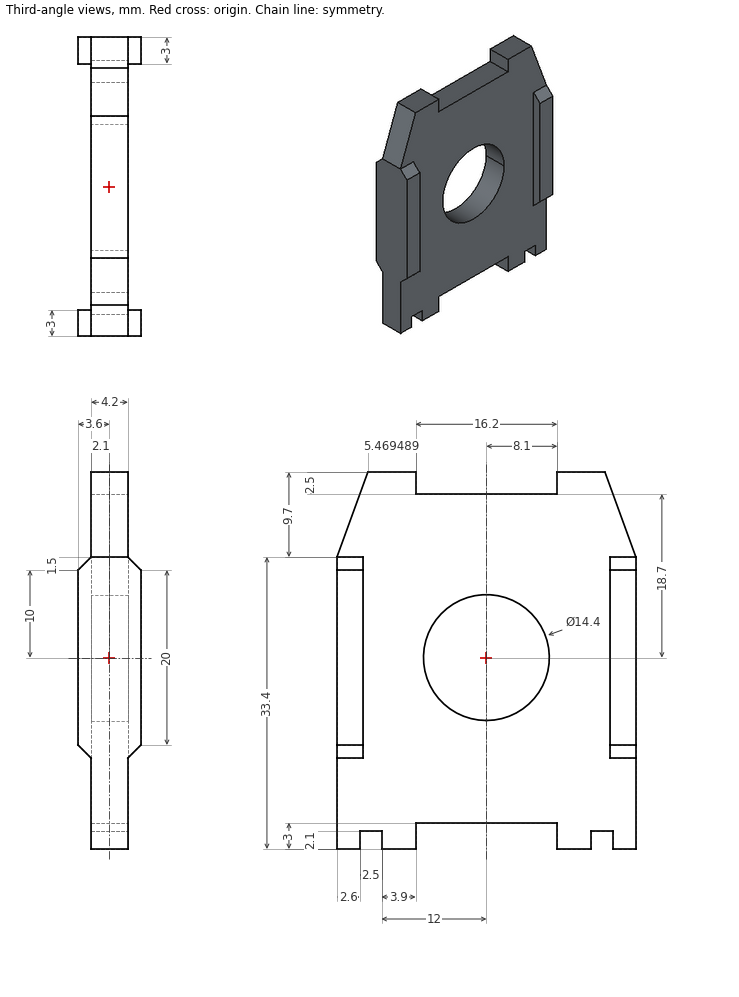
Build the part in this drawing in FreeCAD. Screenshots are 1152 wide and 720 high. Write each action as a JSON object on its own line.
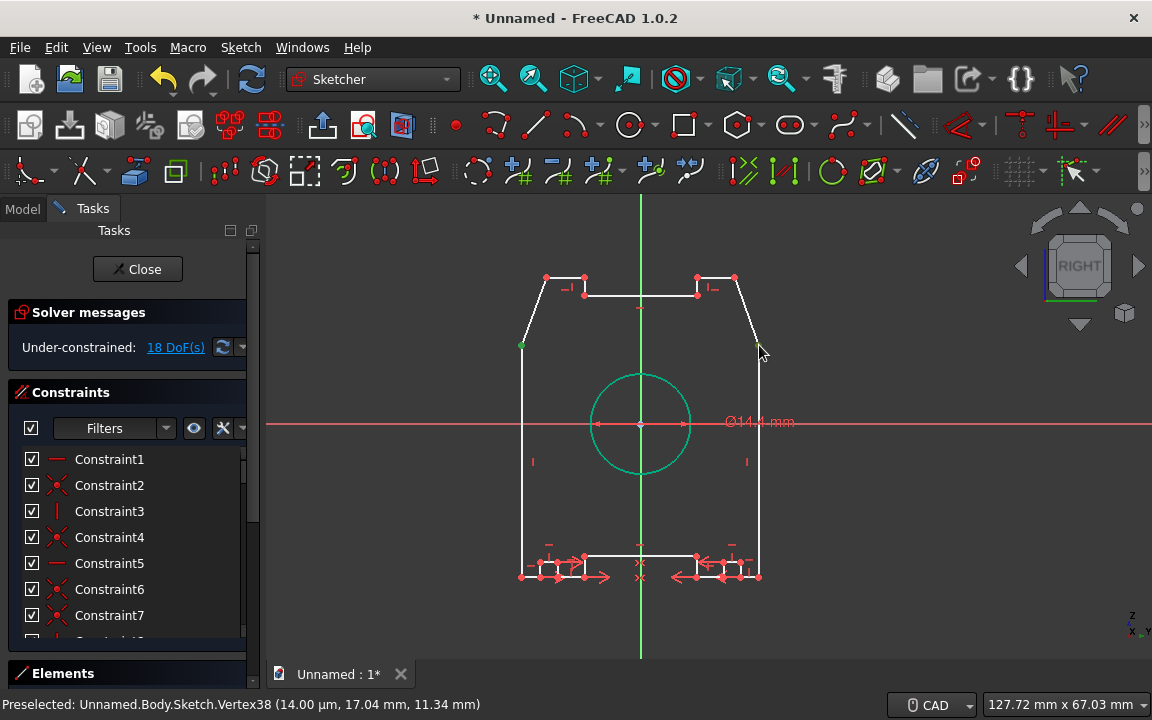
{"action": "left_click", "coordinate": [641, 602]}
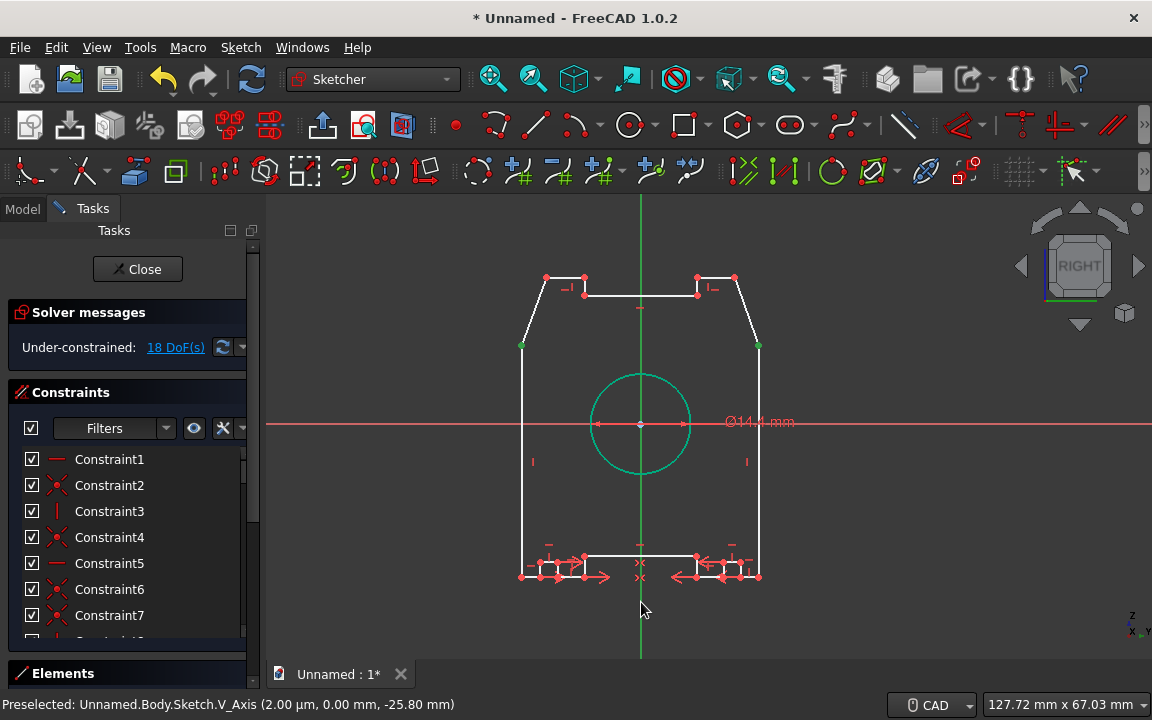
{"action": "key", "text": "s"}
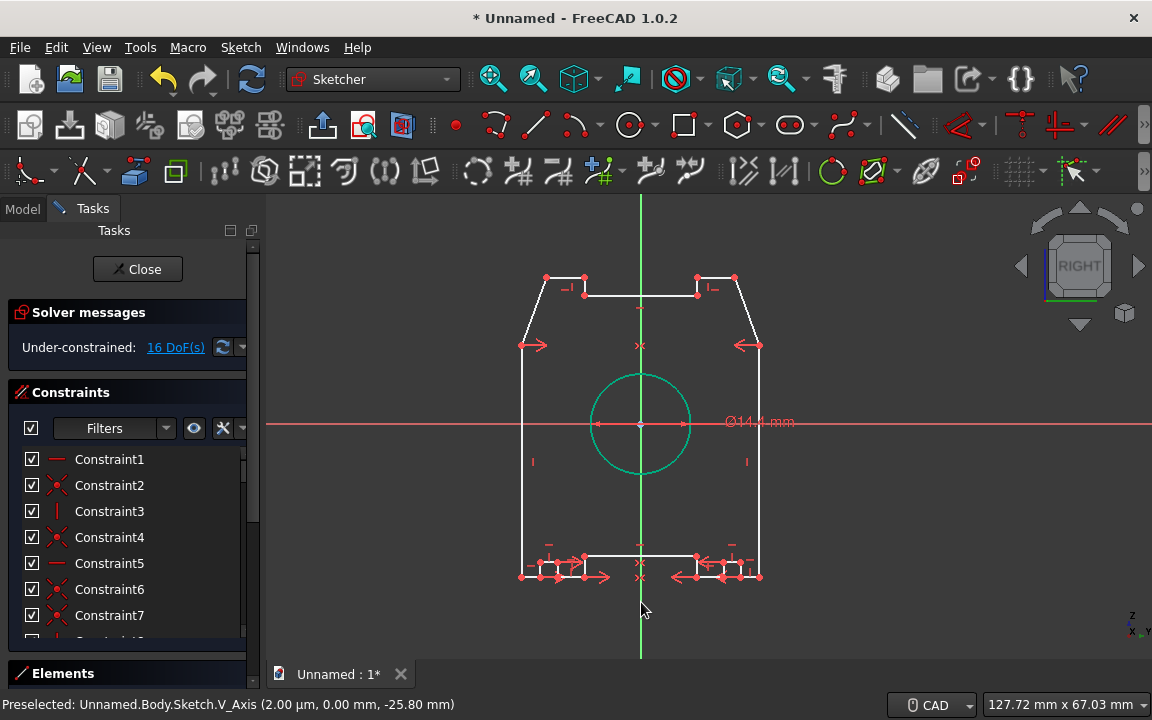
{"action": "left_click", "coordinate": [547, 278]}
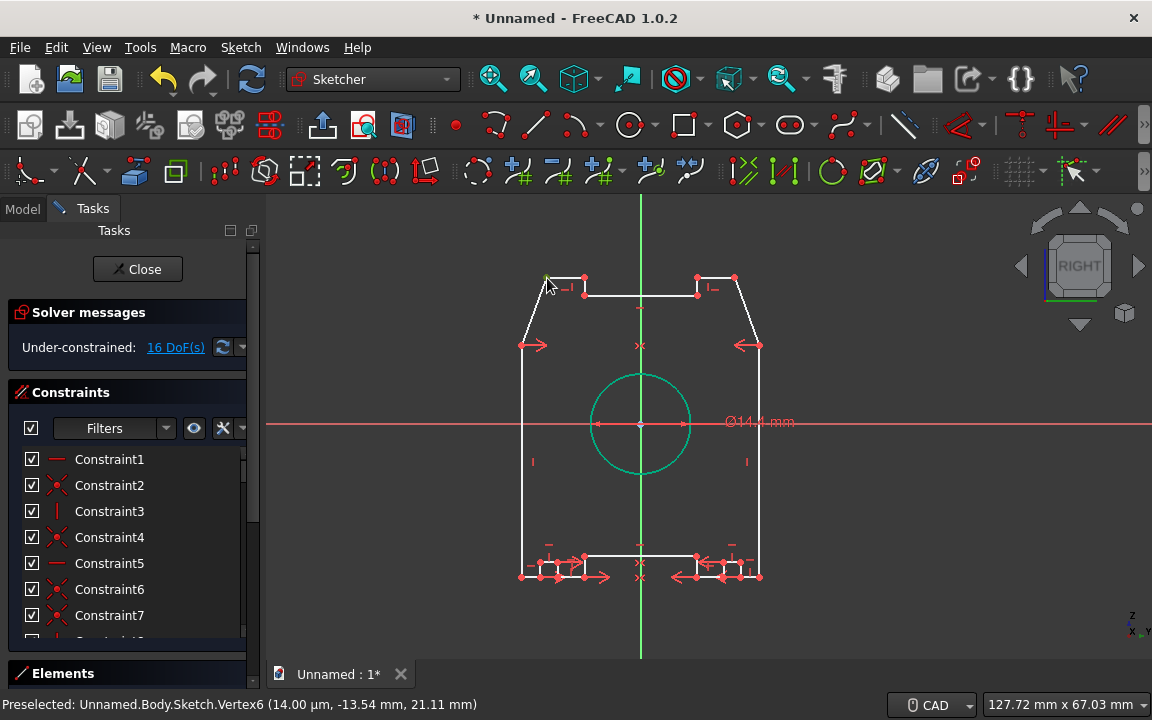
{"action": "left_click", "coordinate": [735, 278]}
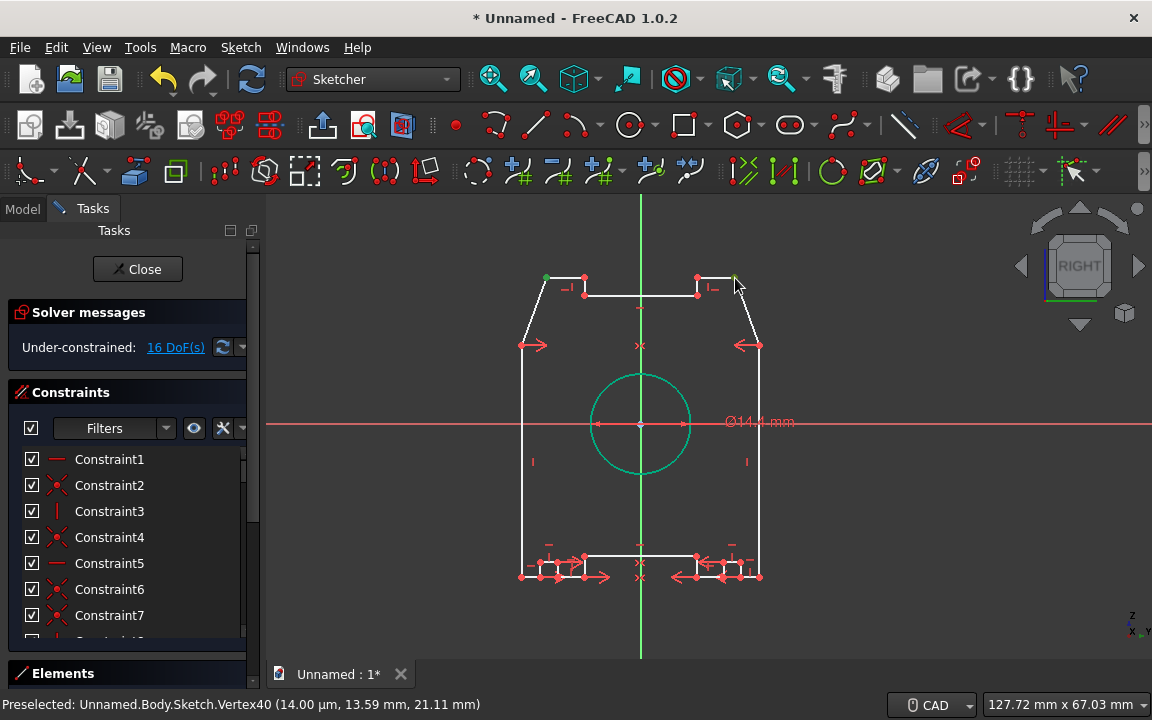
{"action": "left_click", "coordinate": [641, 602]}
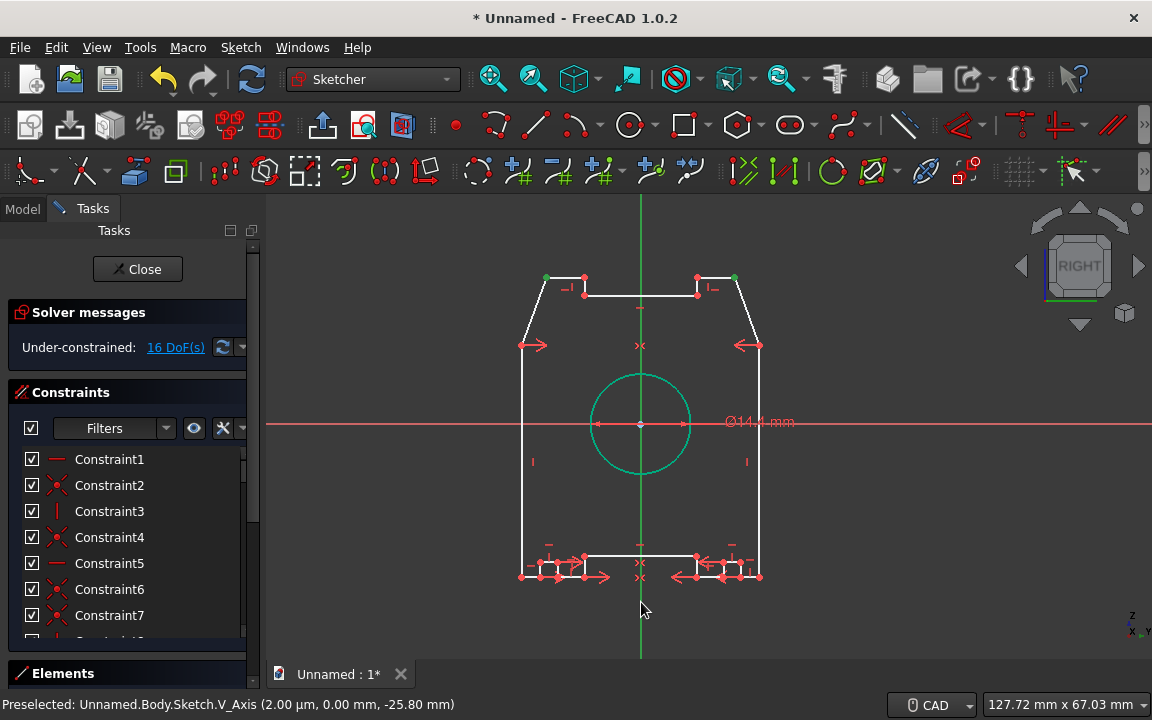
{"action": "key", "text": "s"}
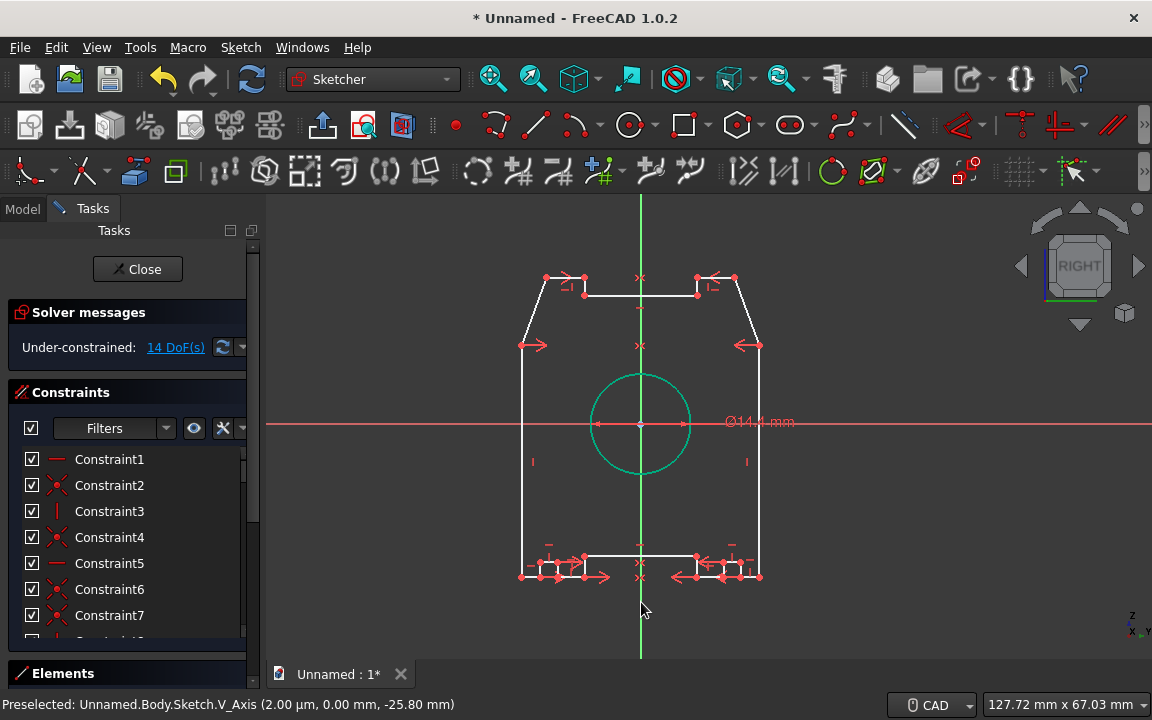
{"action": "key", "text": "d"}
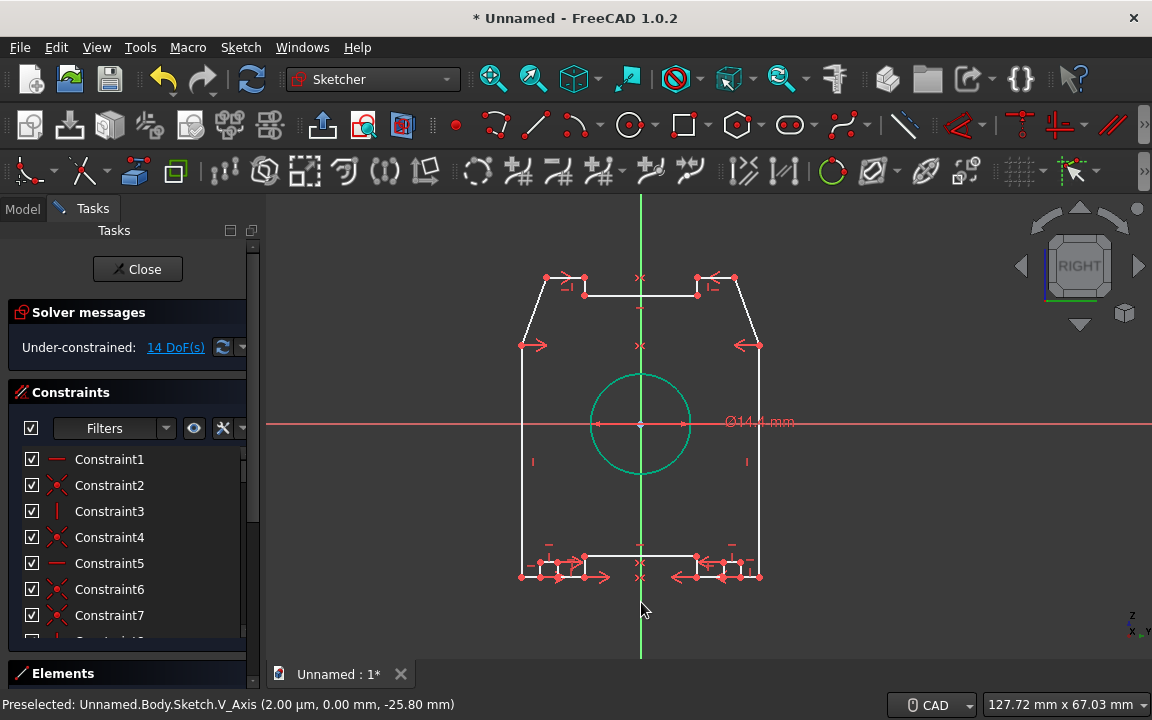
{"action": "scroll", "coordinate": [585, 567], "scroll_direction": "up", "scroll_amount": 4}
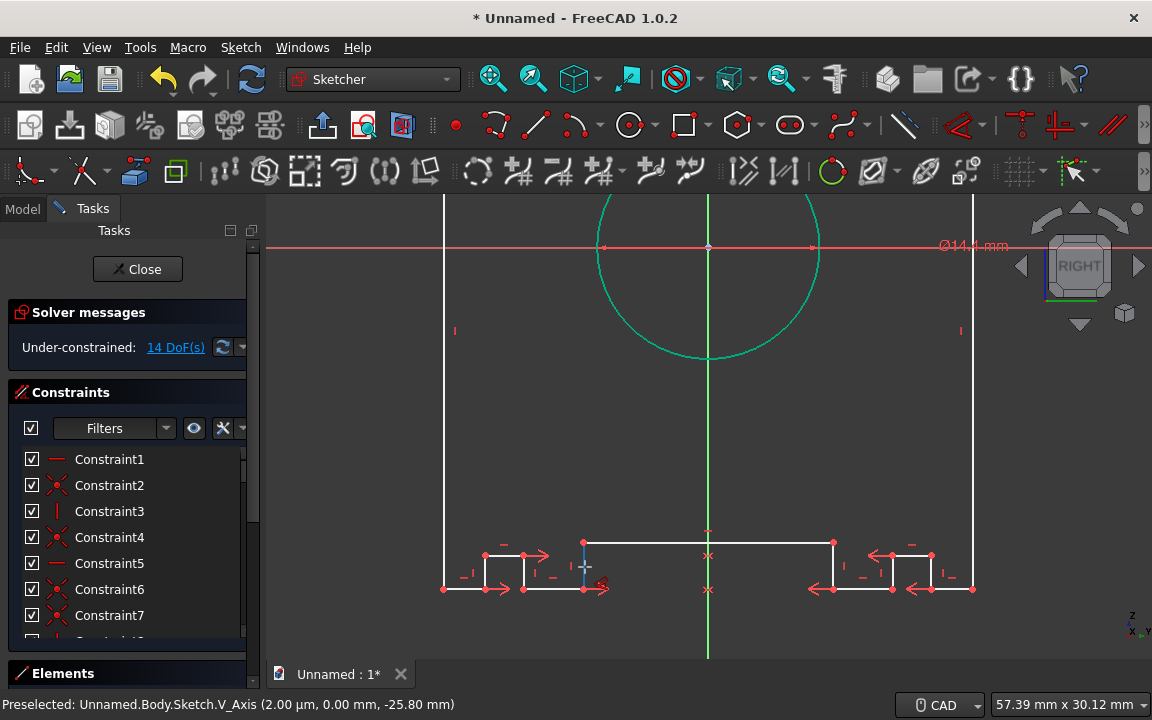
{"action": "left_click", "coordinate": [584, 566]}
{"action": "left_click", "coordinate": [550, 566]}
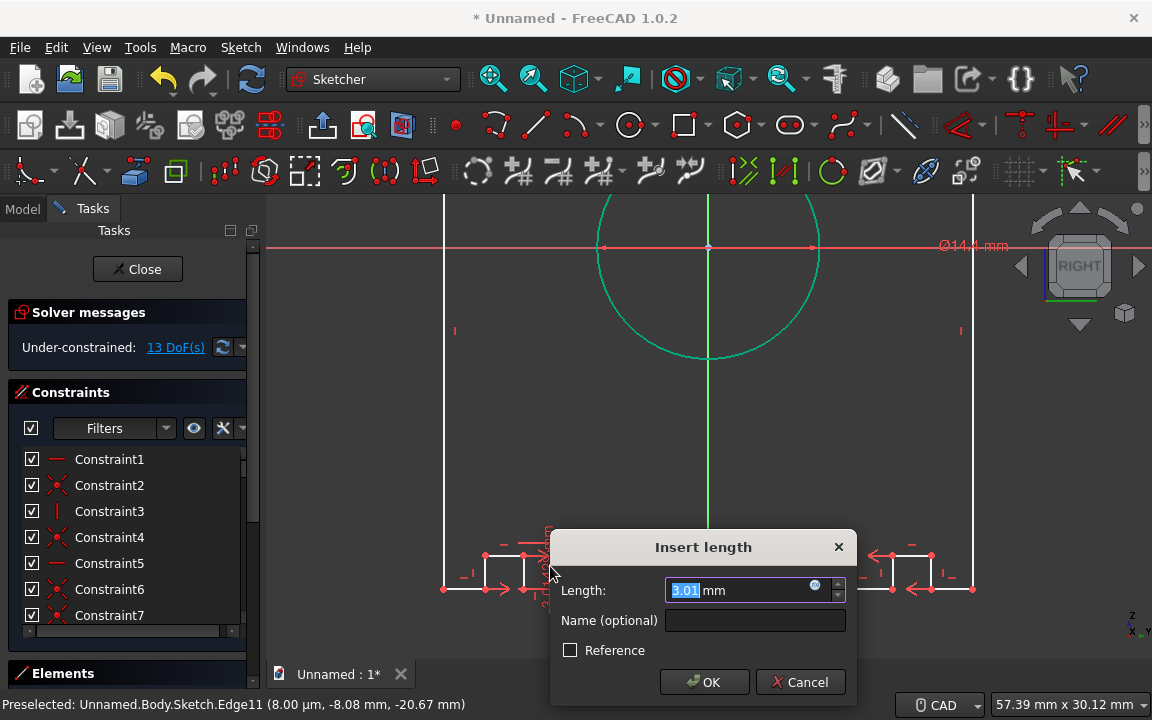
{"action": "type", "text": "3"}
{"action": "key", "text": "Return"}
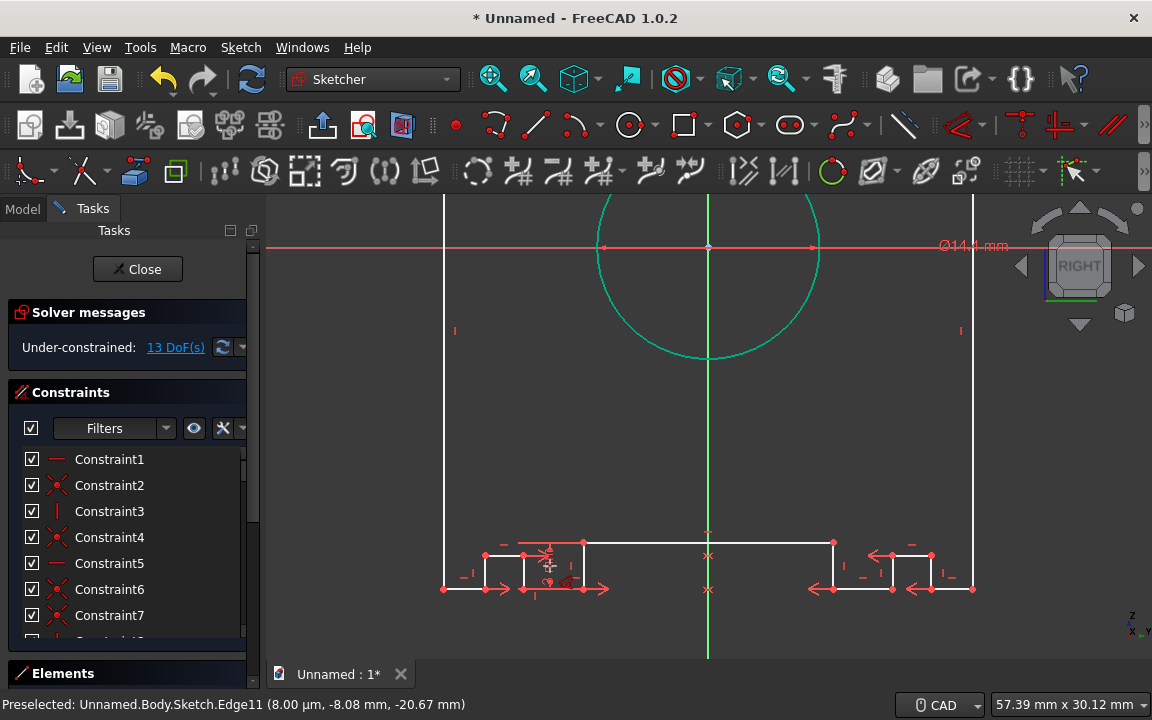
{"action": "scroll", "coordinate": [585, 568], "scroll_direction": "down", "scroll_amount": 4}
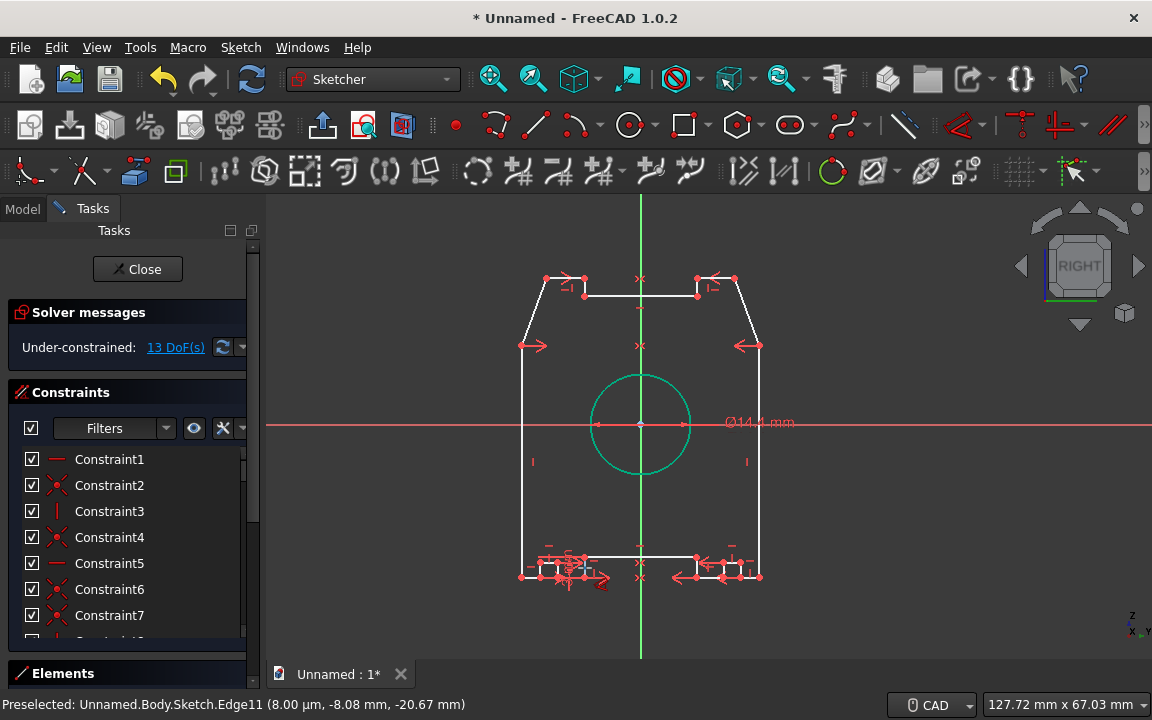
{"action": "scroll", "coordinate": [585, 291], "scroll_direction": "up", "scroll_amount": 5}